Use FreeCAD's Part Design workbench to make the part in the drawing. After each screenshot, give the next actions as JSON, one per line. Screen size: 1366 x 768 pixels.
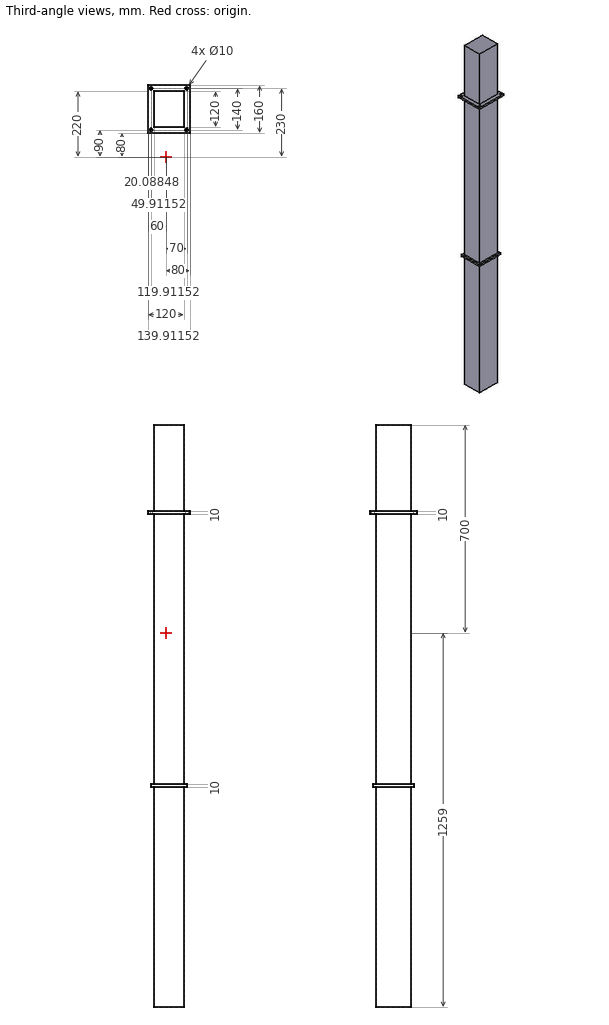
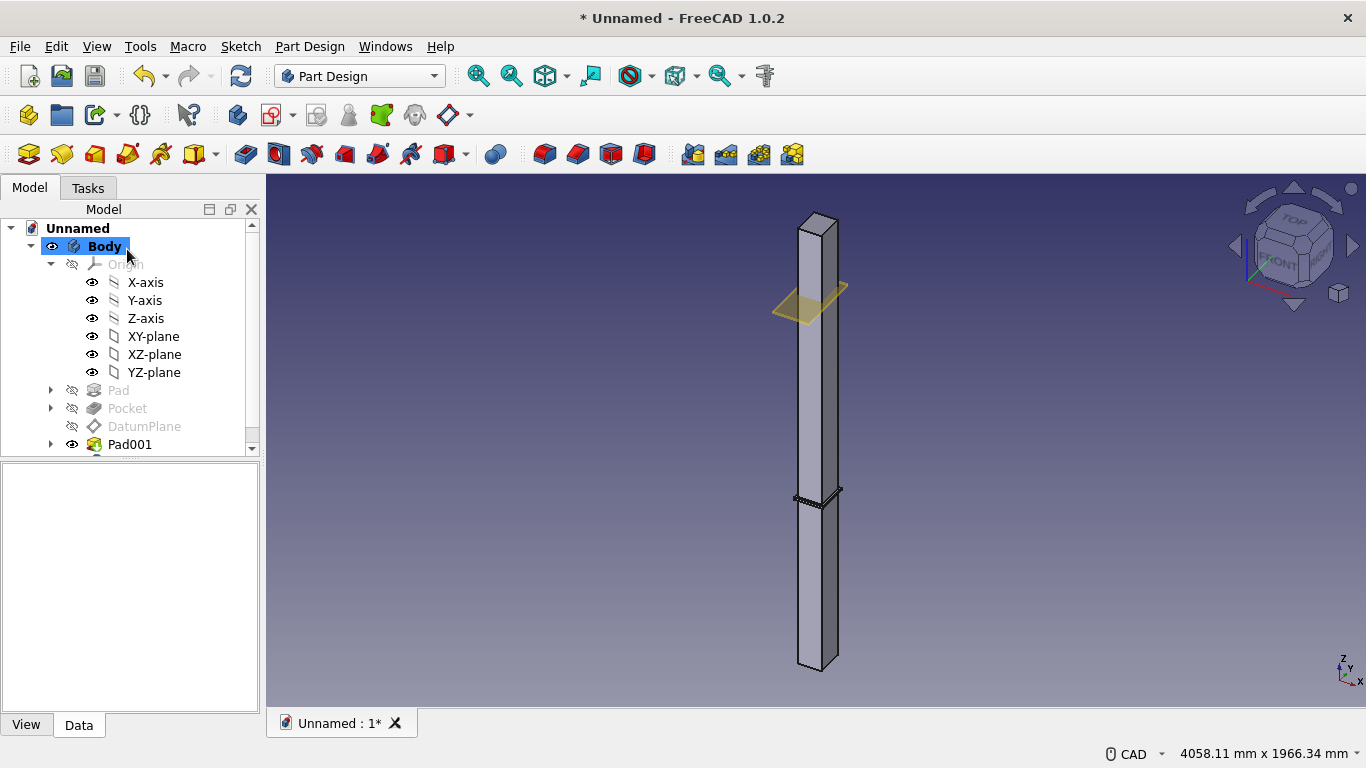
{"action": "scroll", "coordinate": [101, 332], "scroll_direction": "down", "scroll_amount": 3}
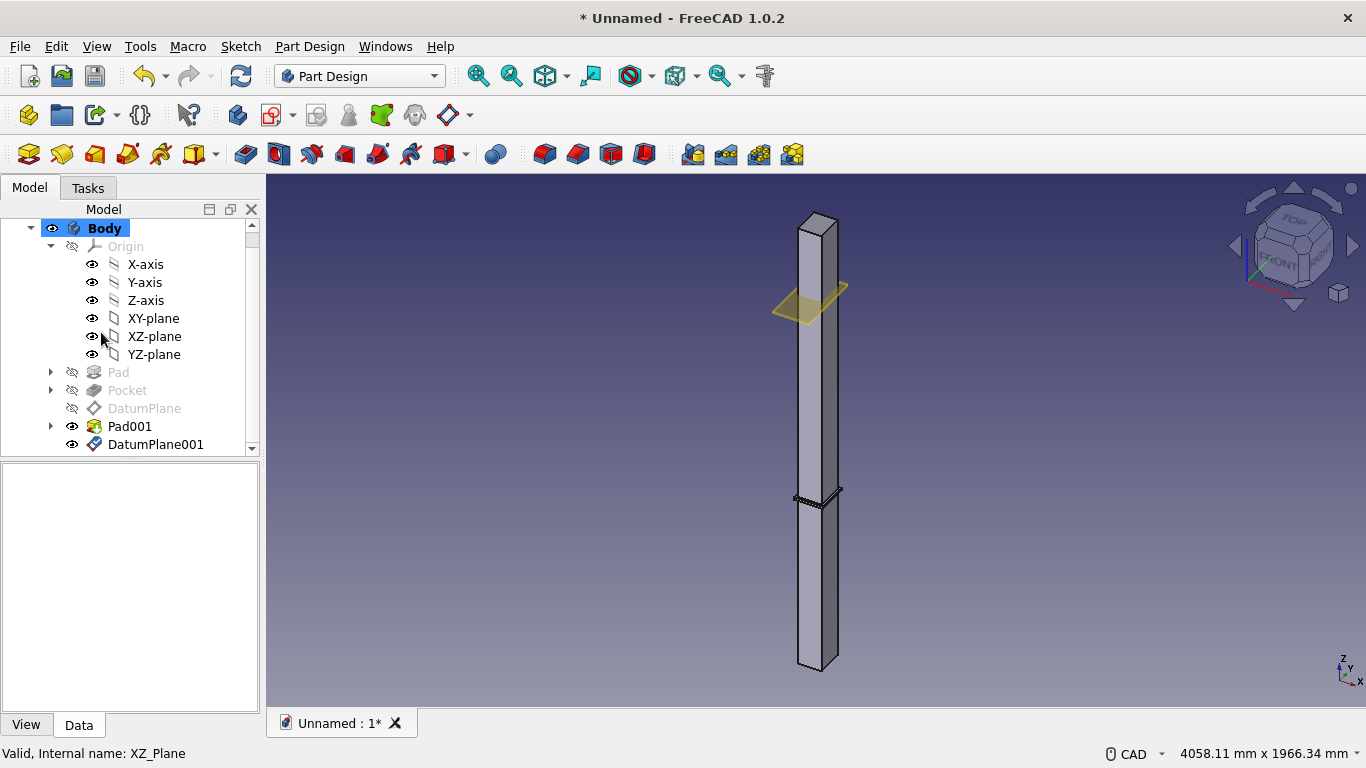
{"action": "left_click", "coordinate": [117, 444]}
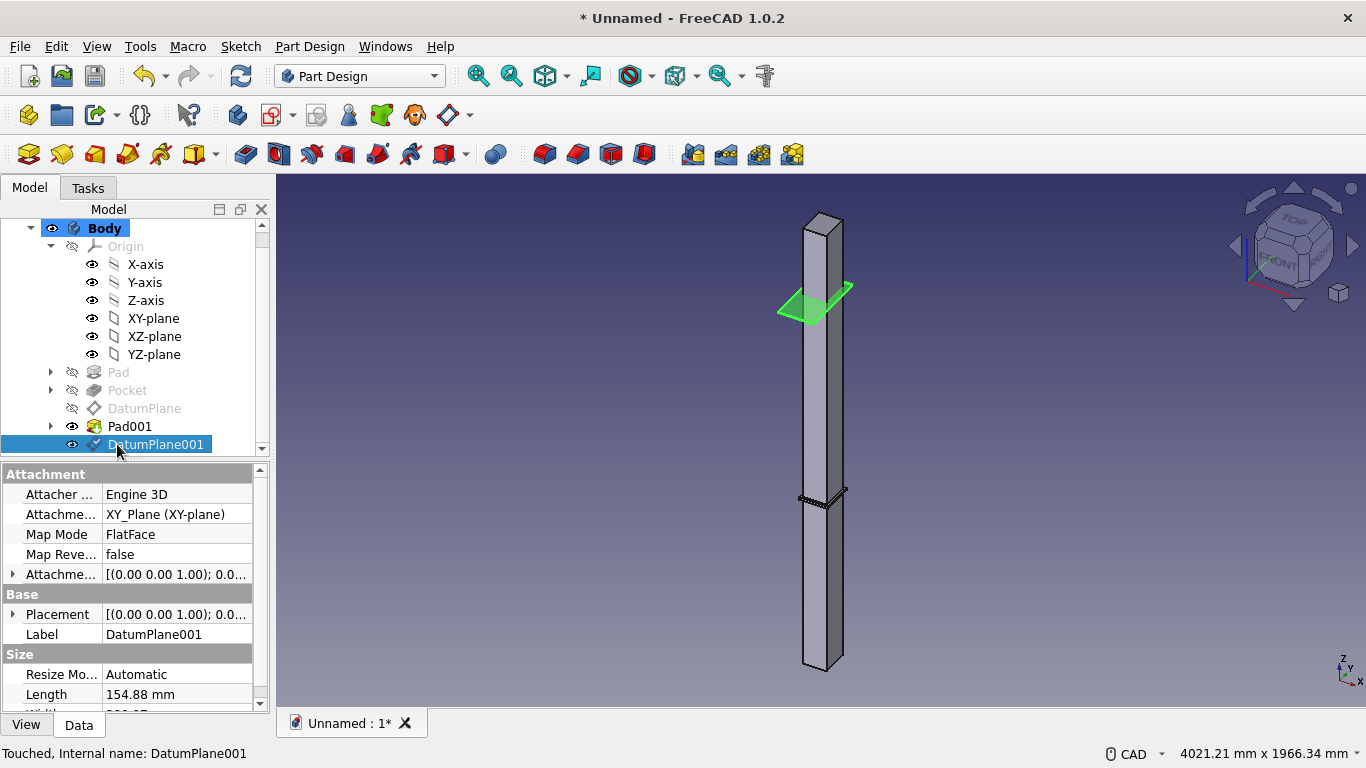
{"action": "left_click", "coordinate": [270, 116]}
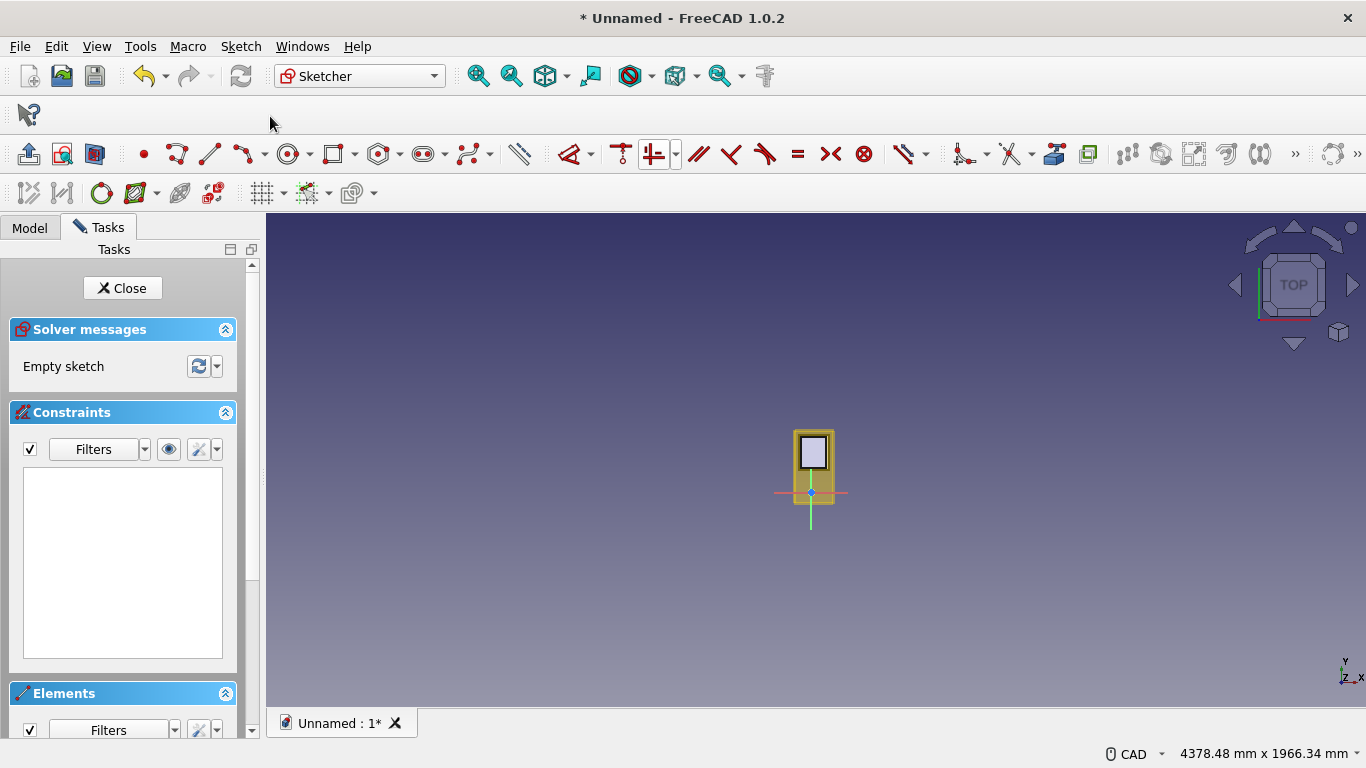
{"action": "key", "text": "q s"}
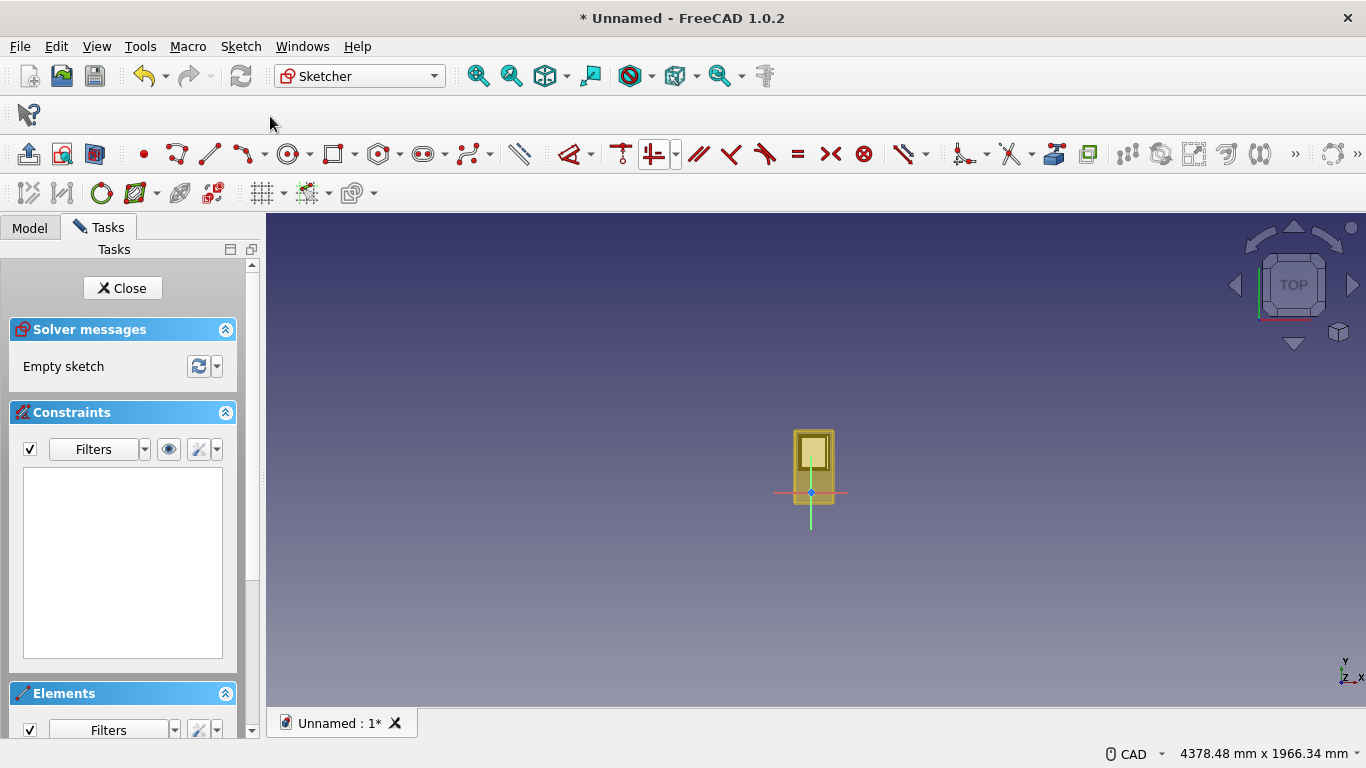
{"action": "scroll", "coordinate": [831, 463], "scroll_direction": "up", "scroll_amount": 8}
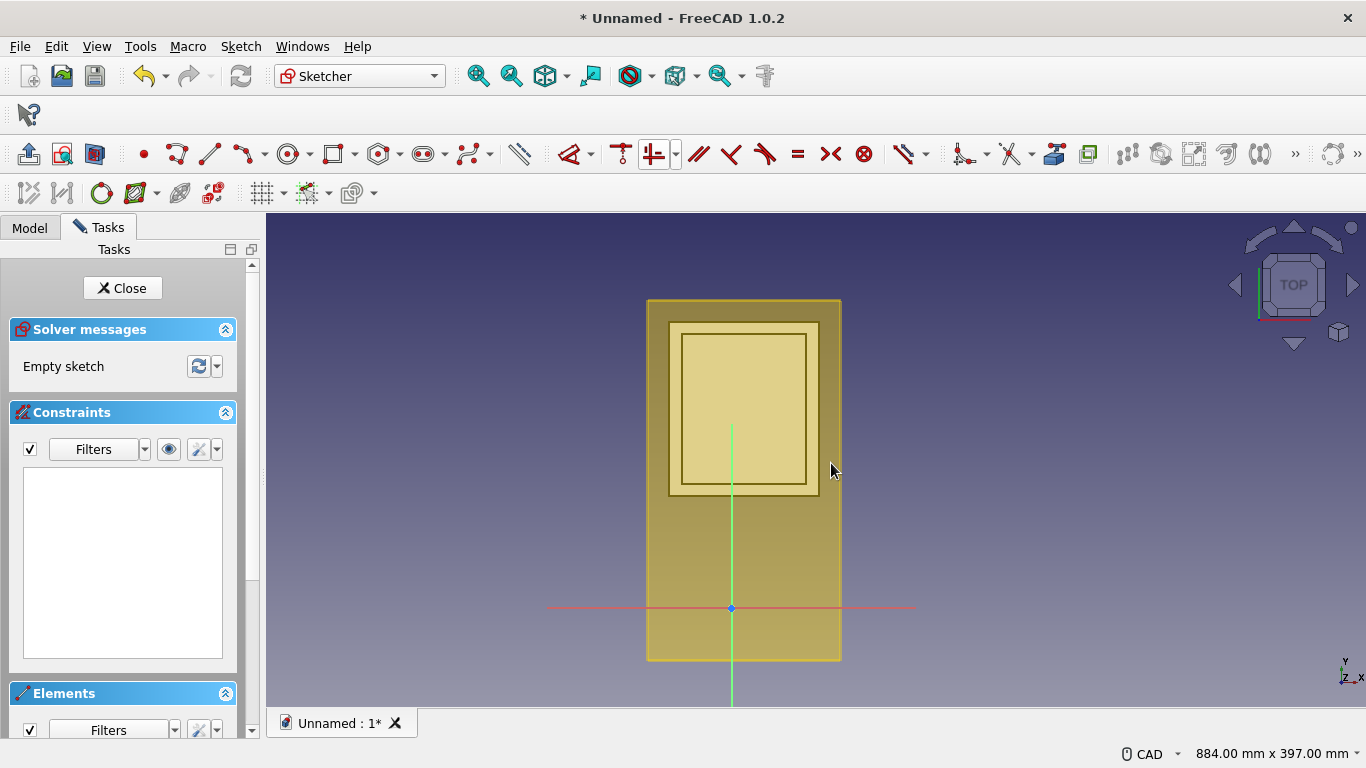
{"action": "key", "text": "g r"}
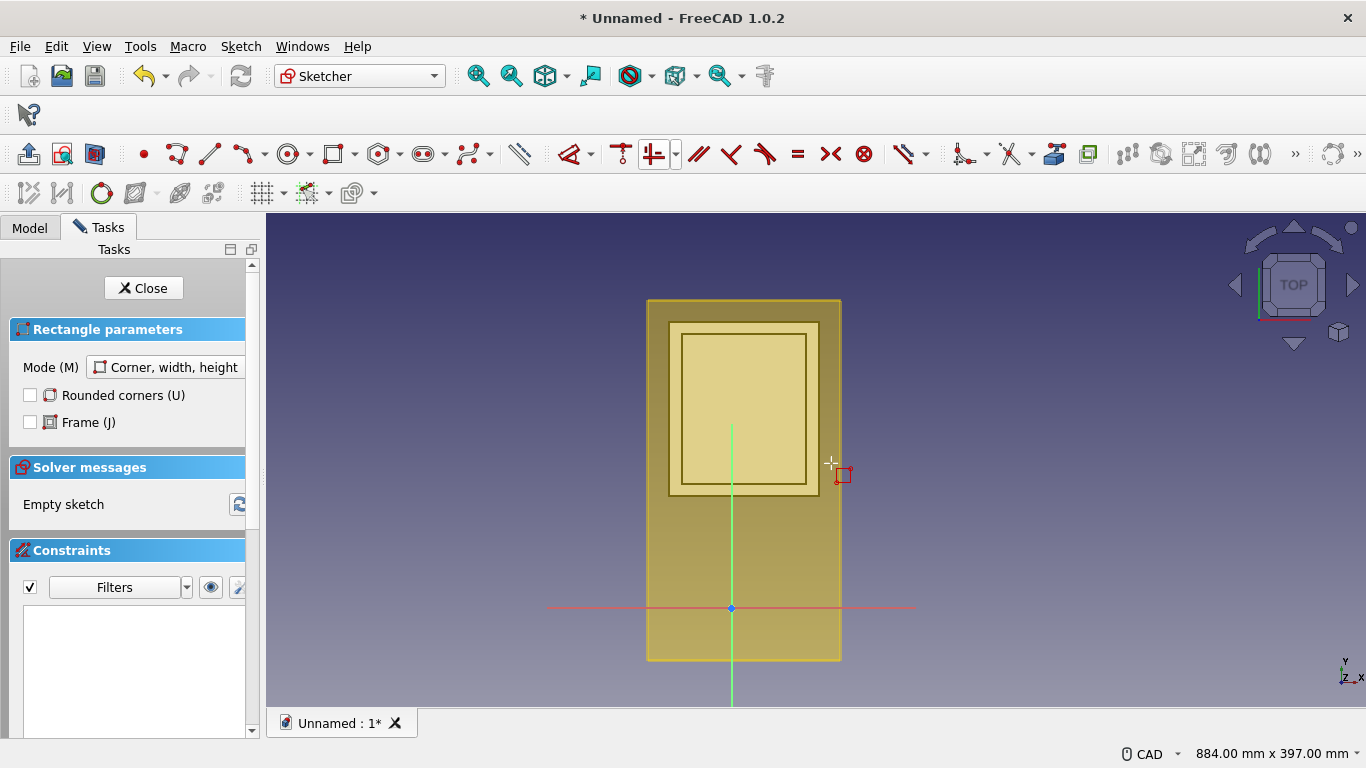
{"action": "left_click", "coordinate": [657, 309]}
{"action": "mouse_move", "coordinate": [831, 509]}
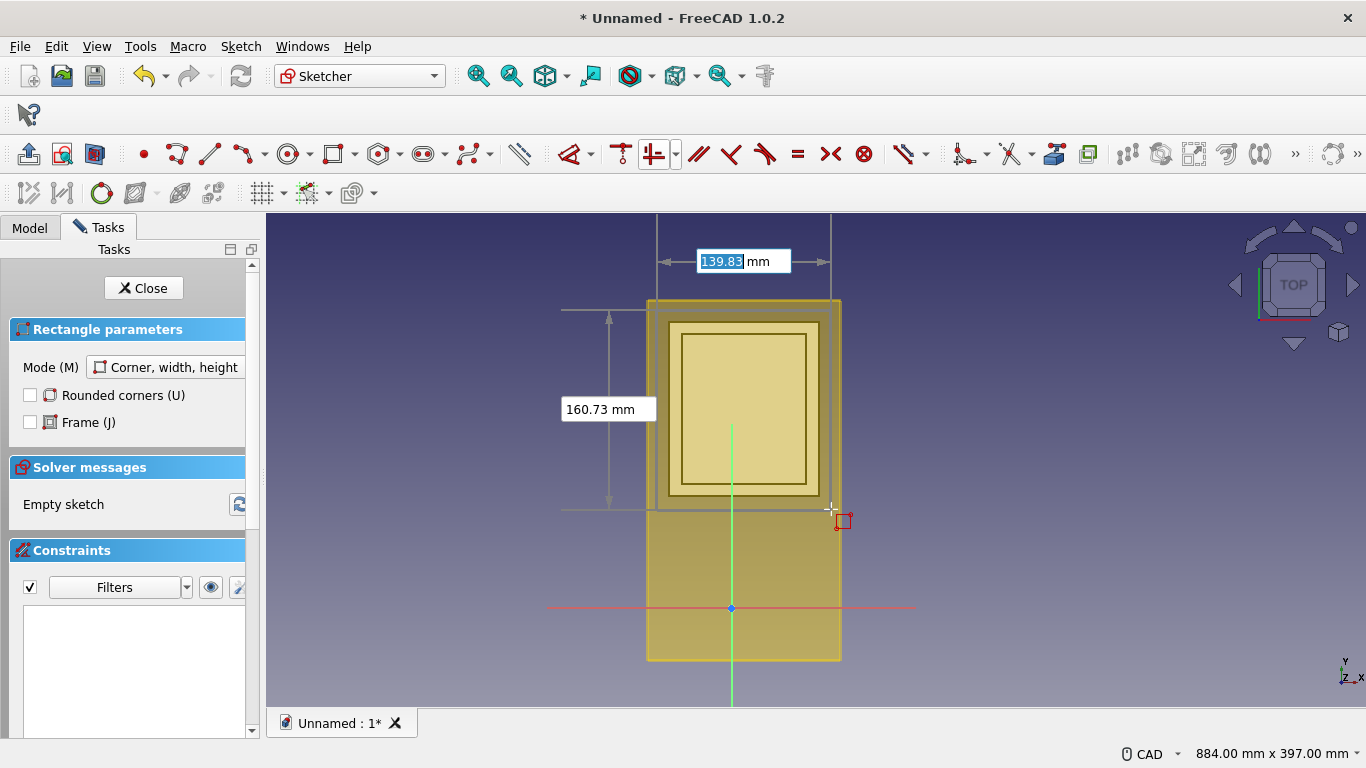
{"action": "type", "text": "139.91152"}
{"action": "key", "text": "Tab"}
{"action": "type", "text": "160"}
{"action": "key", "text": "Return"}
{"action": "key", "text": "Escape"}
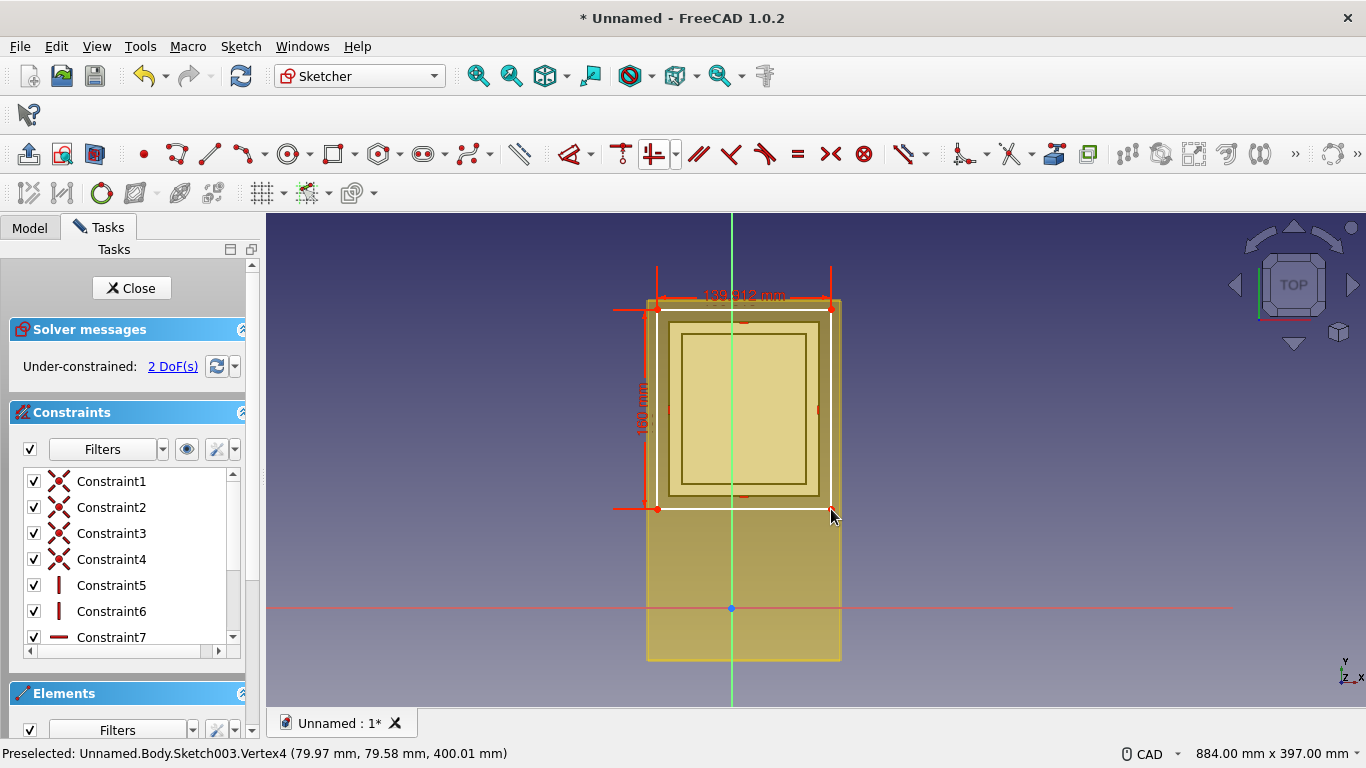
{"action": "key", "text": "d"}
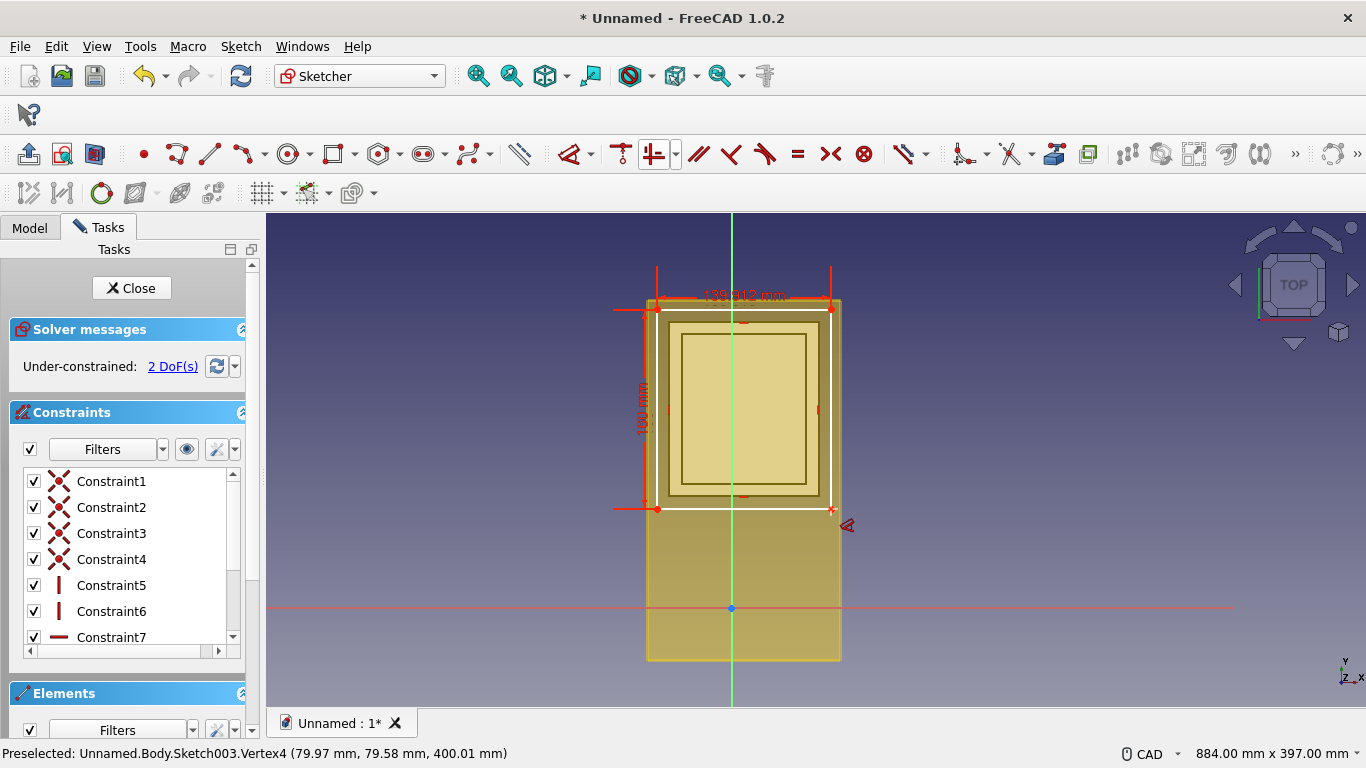
{"action": "left_click", "coordinate": [657, 509]}
{"action": "left_click", "coordinate": [623, 559]}